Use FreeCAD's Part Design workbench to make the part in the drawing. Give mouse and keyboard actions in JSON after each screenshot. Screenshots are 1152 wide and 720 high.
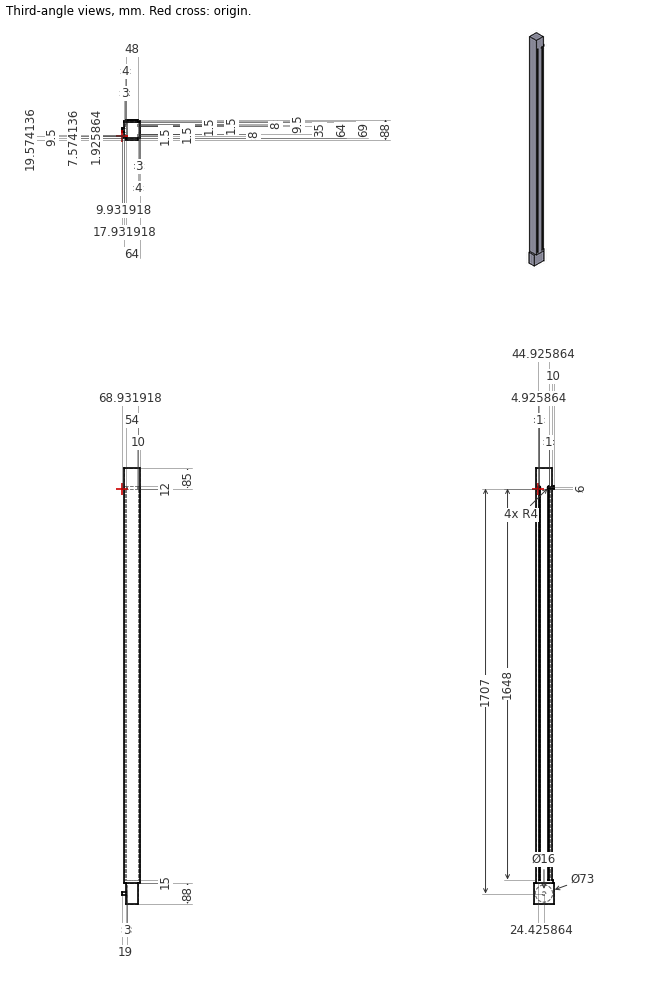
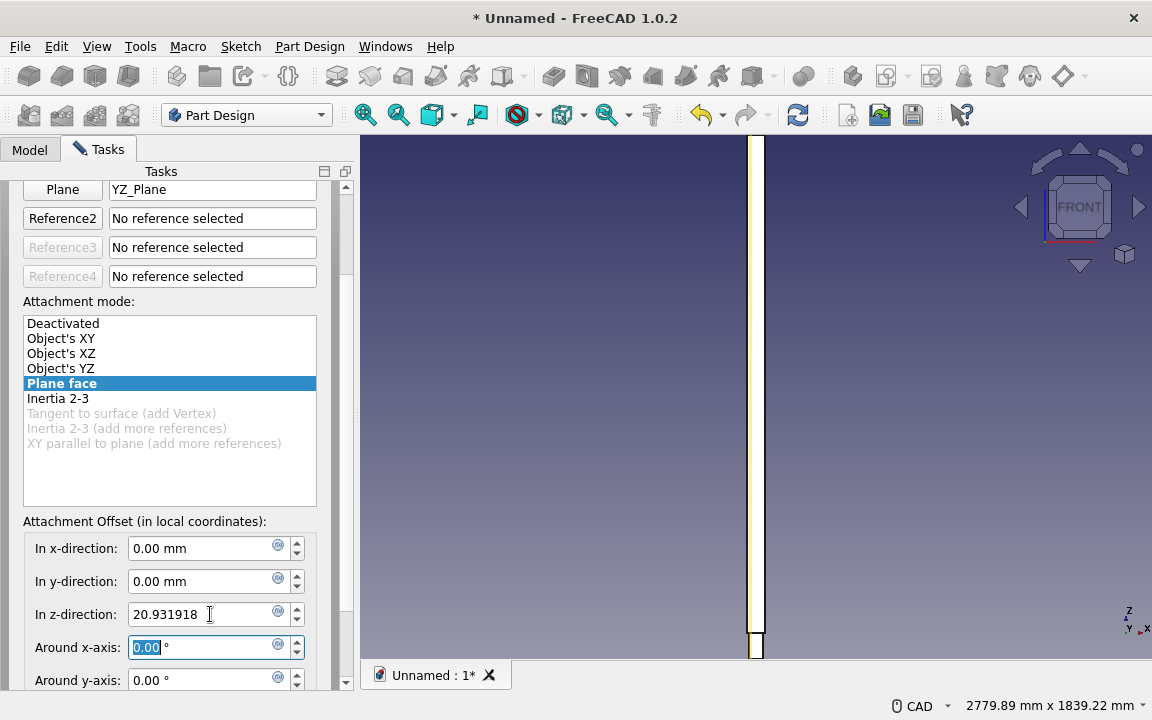
{"action": "scroll", "coordinate": [346, 436], "scroll_direction": "up", "scroll_amount": 3}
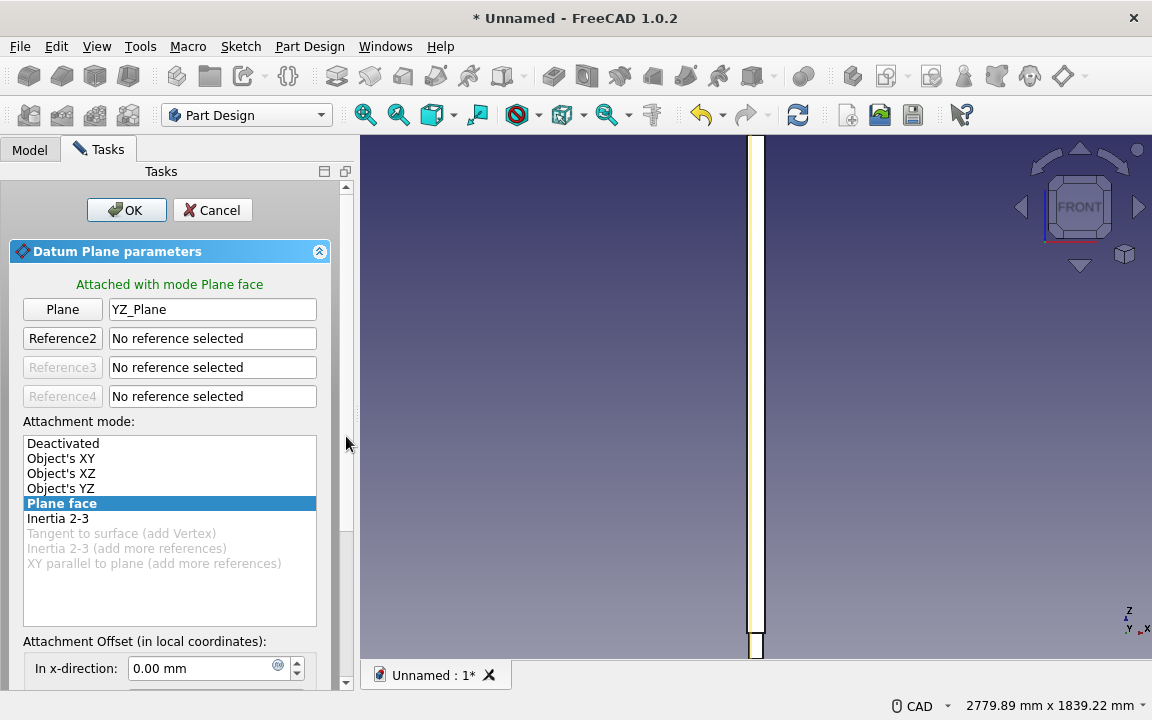
{"action": "left_click", "coordinate": [127, 210]}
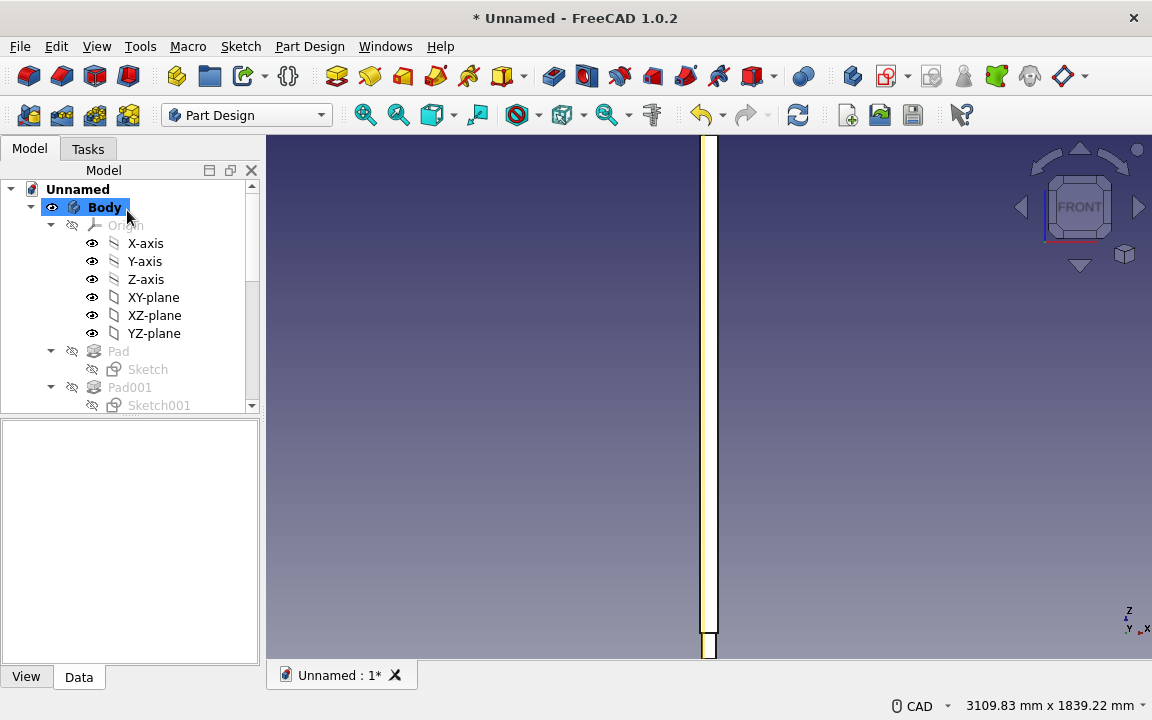
{"action": "scroll", "coordinate": [101, 293], "scroll_direction": "down", "scroll_amount": 3}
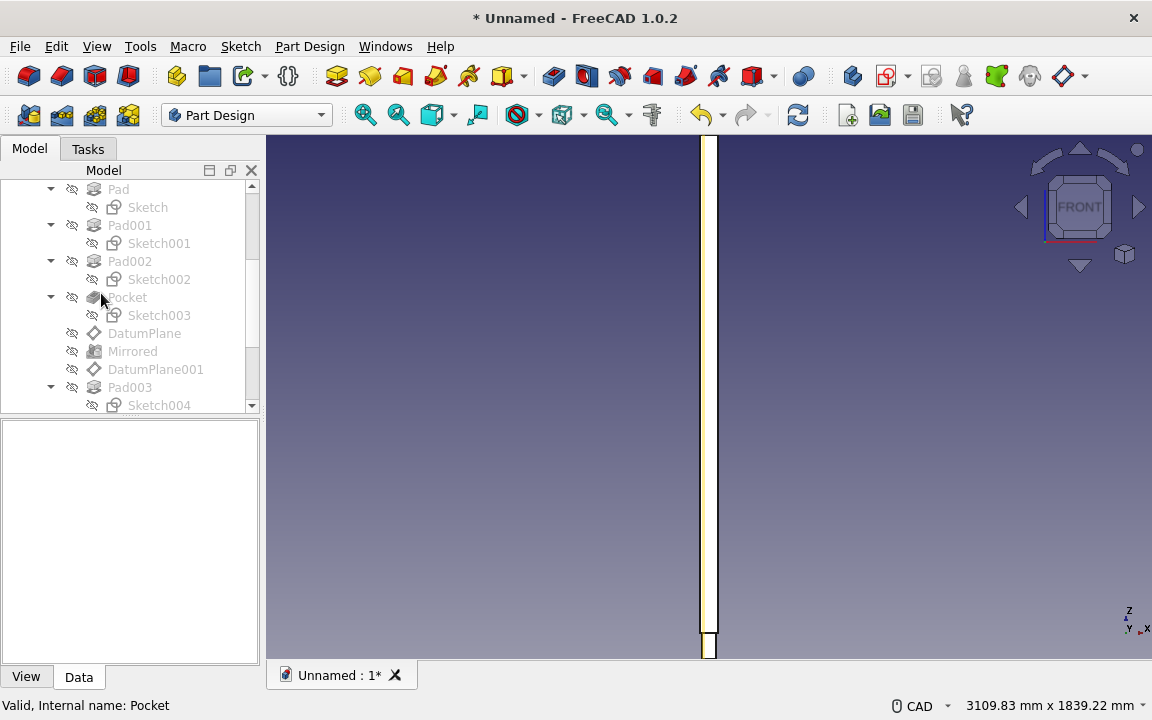
{"action": "scroll", "coordinate": [141, 293], "scroll_direction": "up", "scroll_amount": 15}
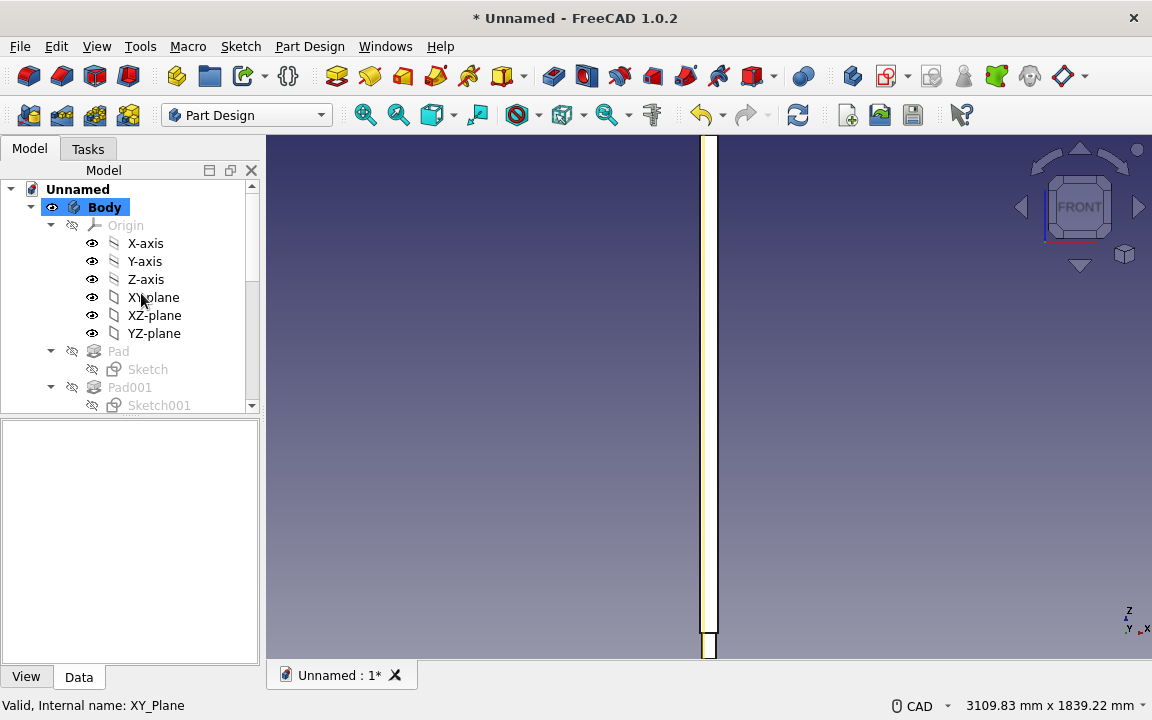
{"action": "scroll", "coordinate": [101, 293], "scroll_direction": "down", "scroll_amount": 6}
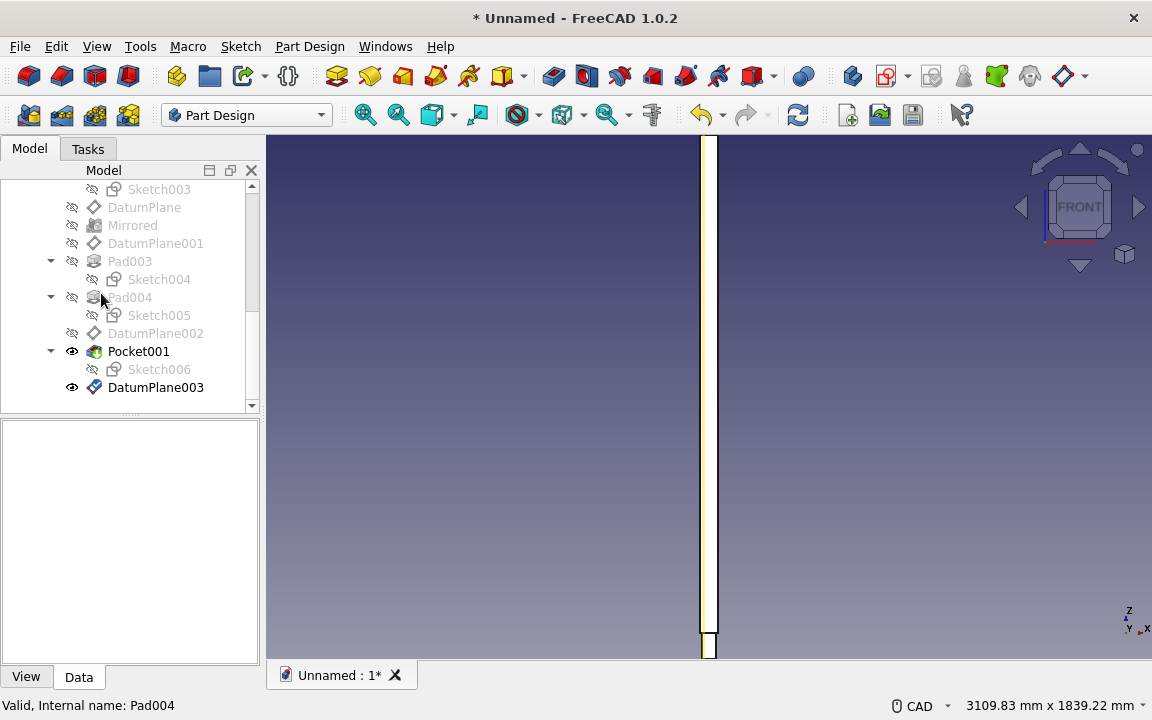
{"action": "left_click", "coordinate": [117, 387]}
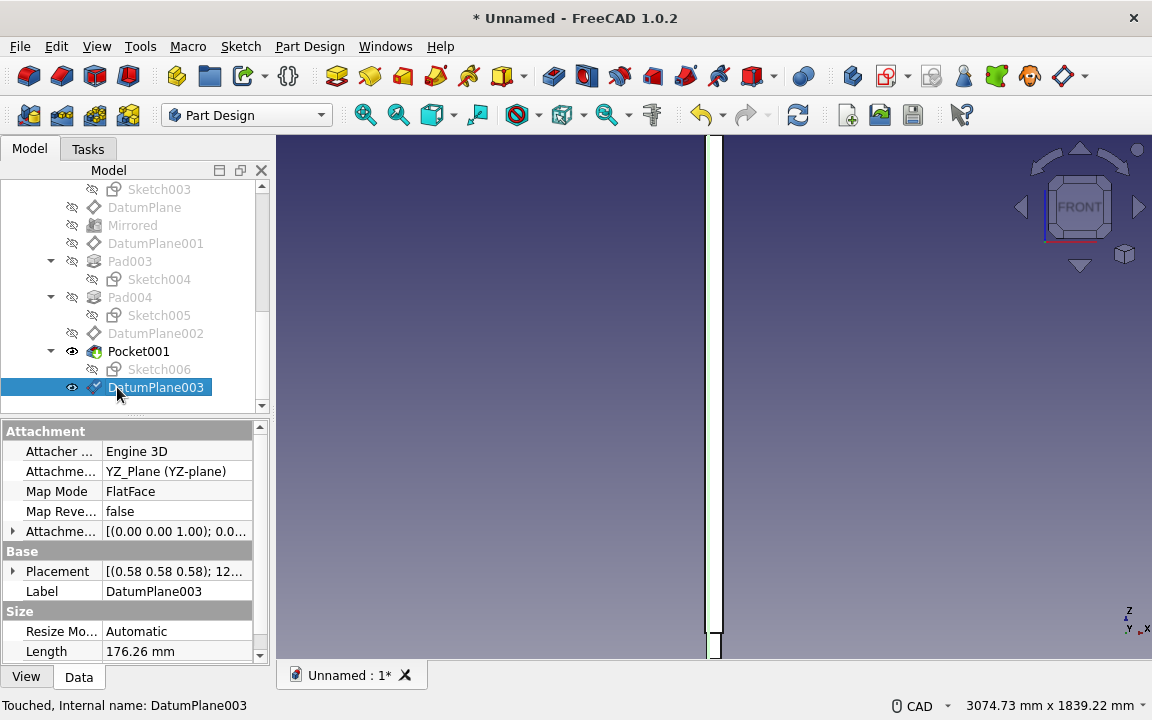
{"action": "left_click", "coordinate": [886, 76]}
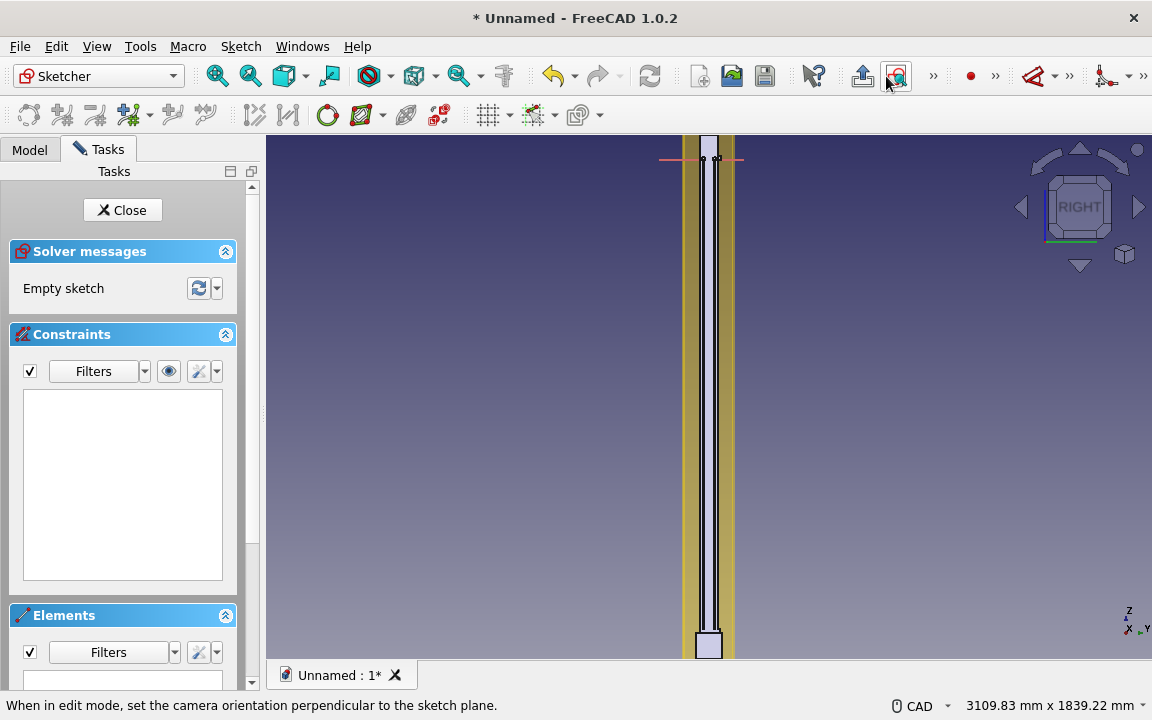
{"action": "key", "text": "q s"}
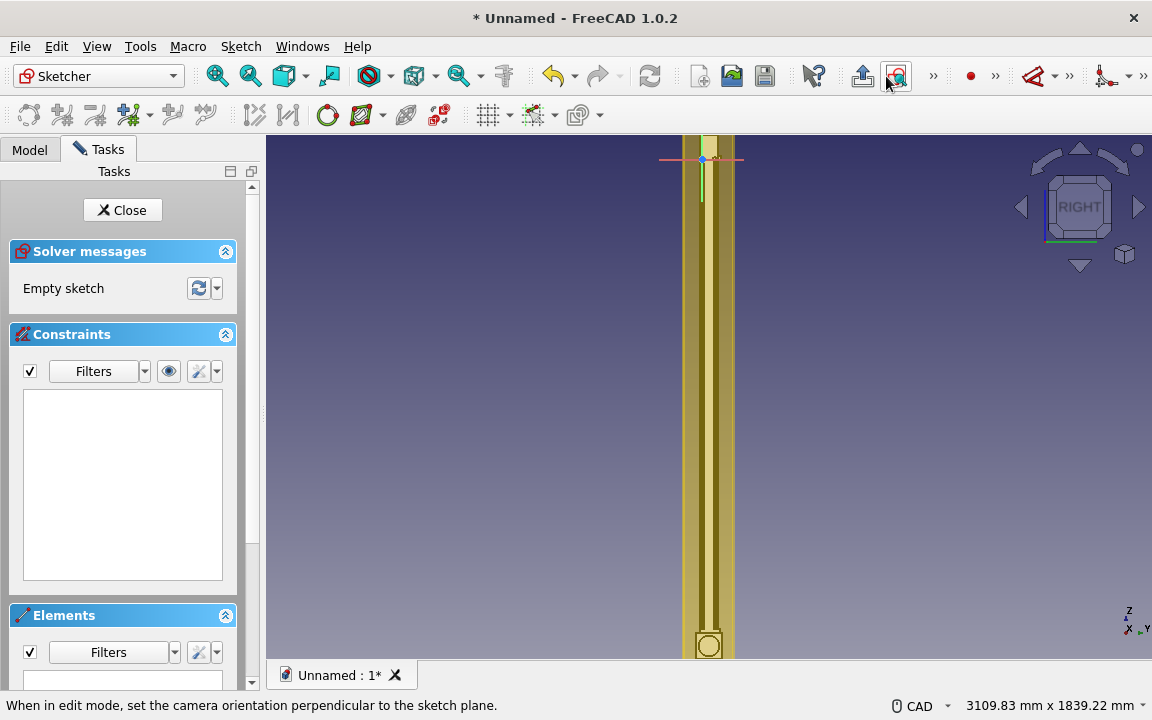
{"action": "scroll", "coordinate": [640, 397], "scroll_direction": "down", "scroll_amount": 5}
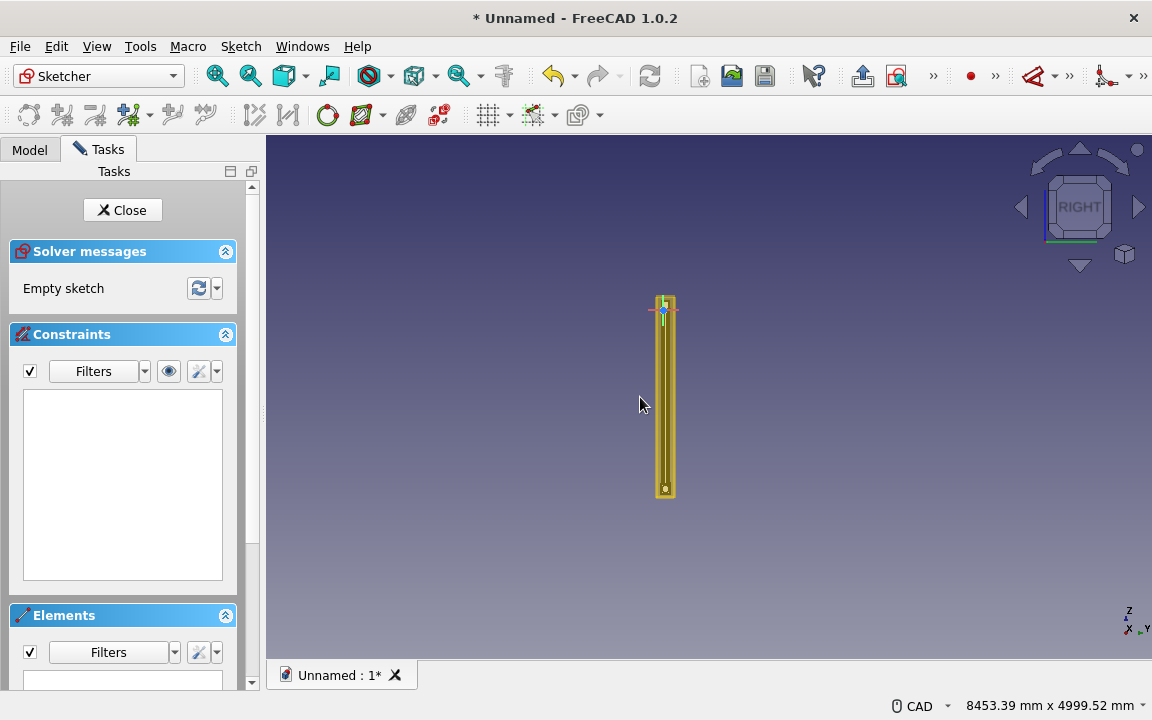
{"action": "scroll", "coordinate": [667, 494], "scroll_direction": "up", "scroll_amount": 15}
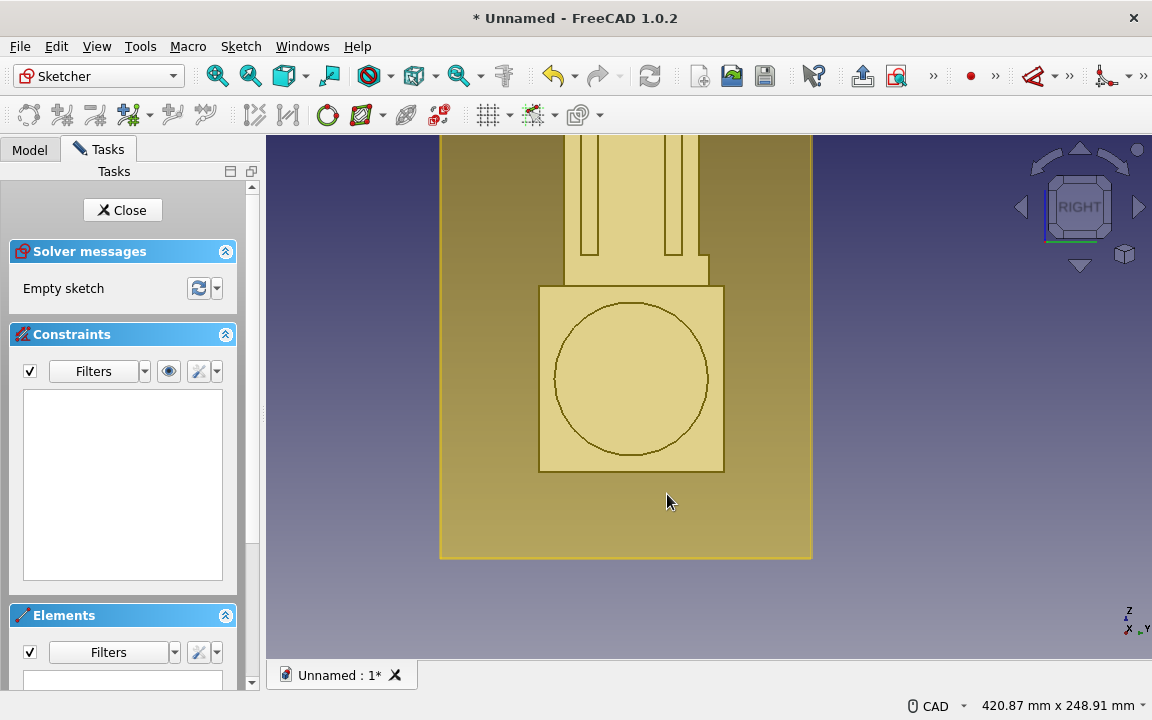
{"action": "scroll", "coordinate": [630, 377], "scroll_direction": "up", "scroll_amount": 11}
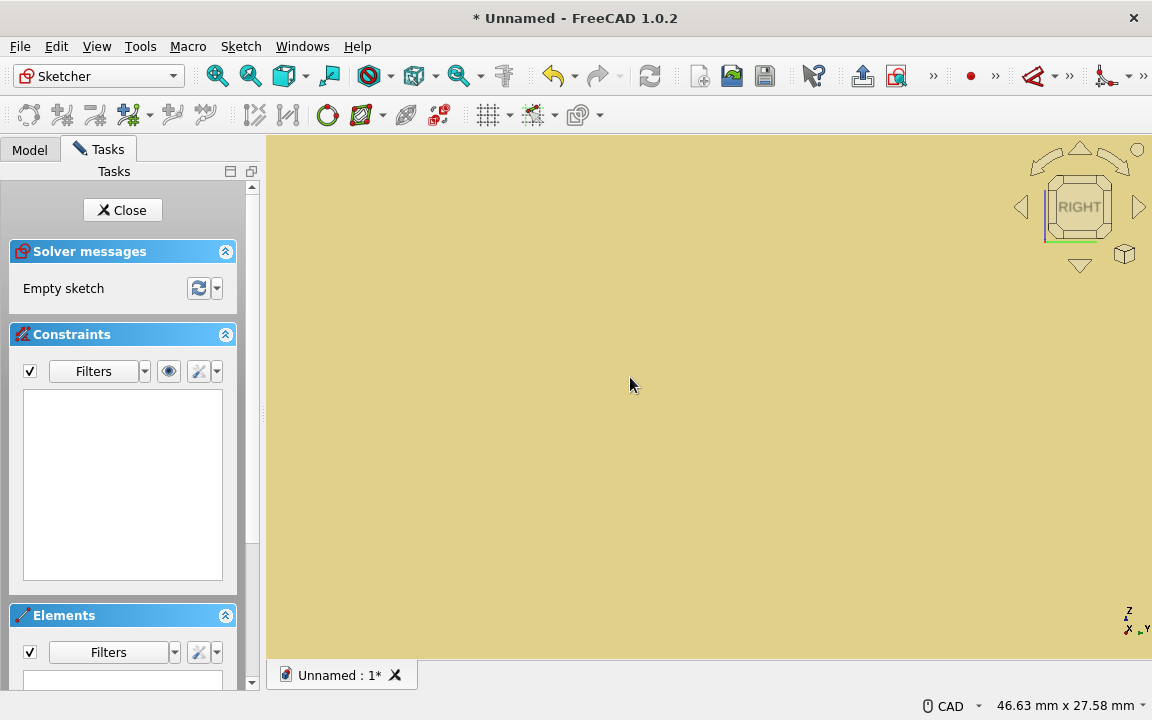
{"action": "key", "text": "g c"}